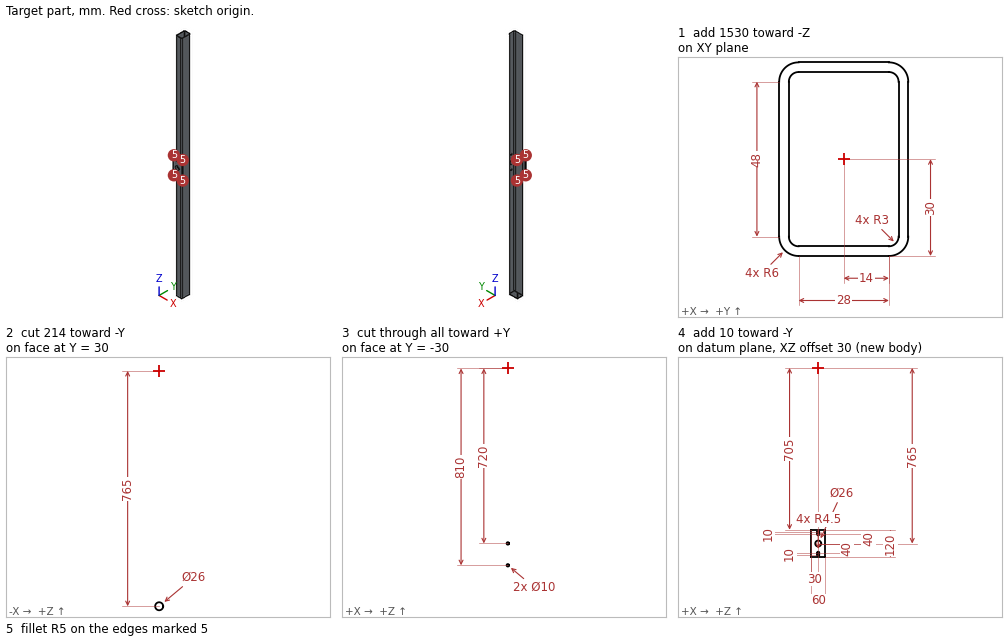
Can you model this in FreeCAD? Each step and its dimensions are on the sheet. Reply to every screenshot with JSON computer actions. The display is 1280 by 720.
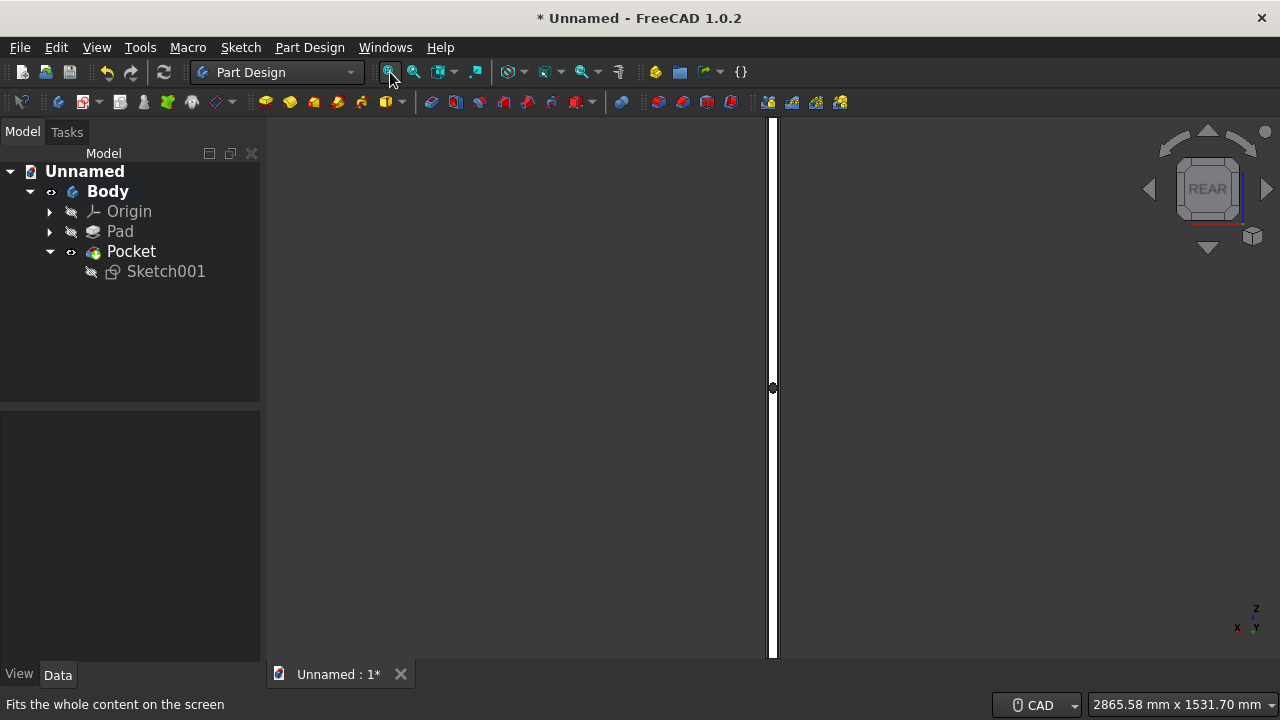
{"action": "key", "text": "0"}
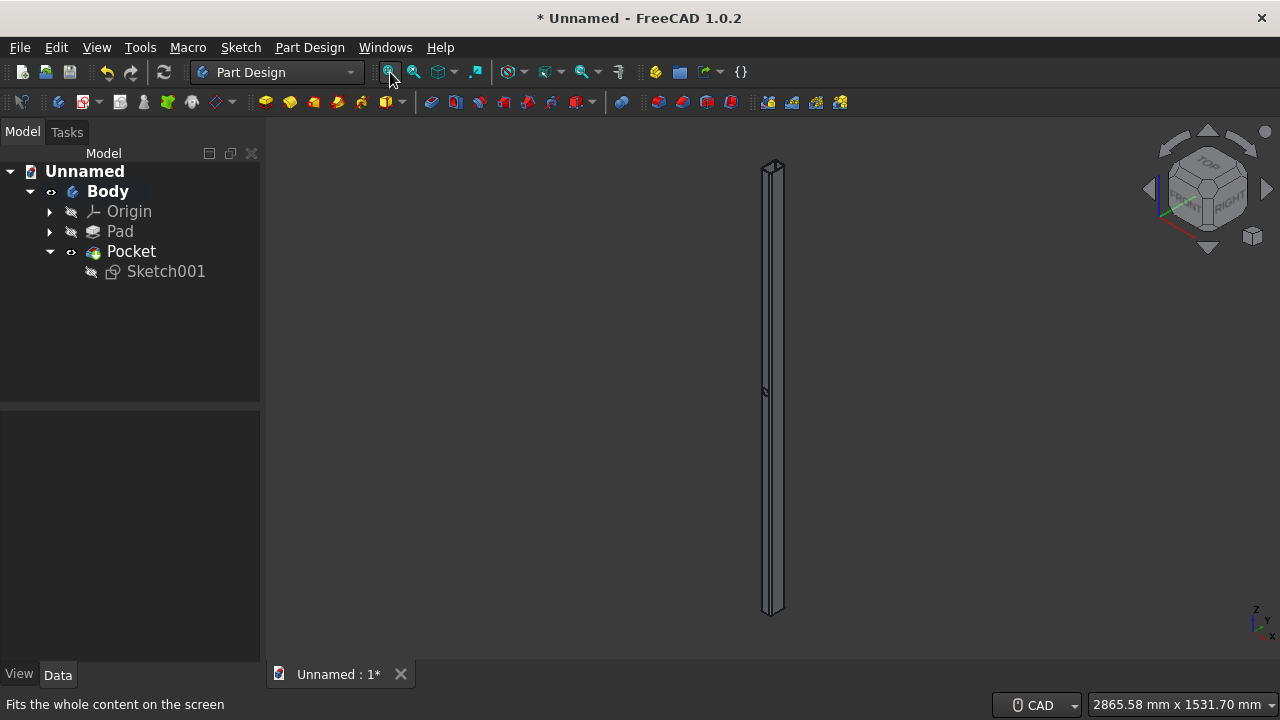
{"action": "scroll", "coordinate": [765, 202], "scroll_direction": "up", "scroll_amount": 5}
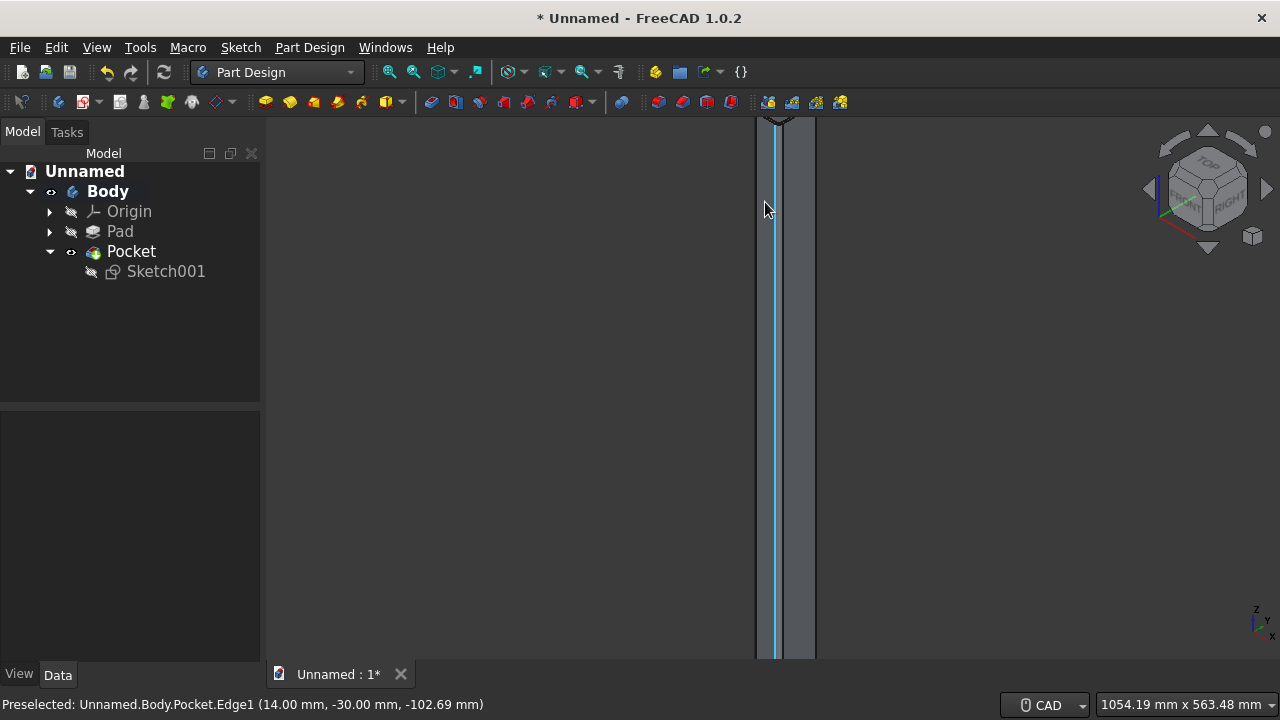
{"action": "left_click", "coordinate": [765, 203]}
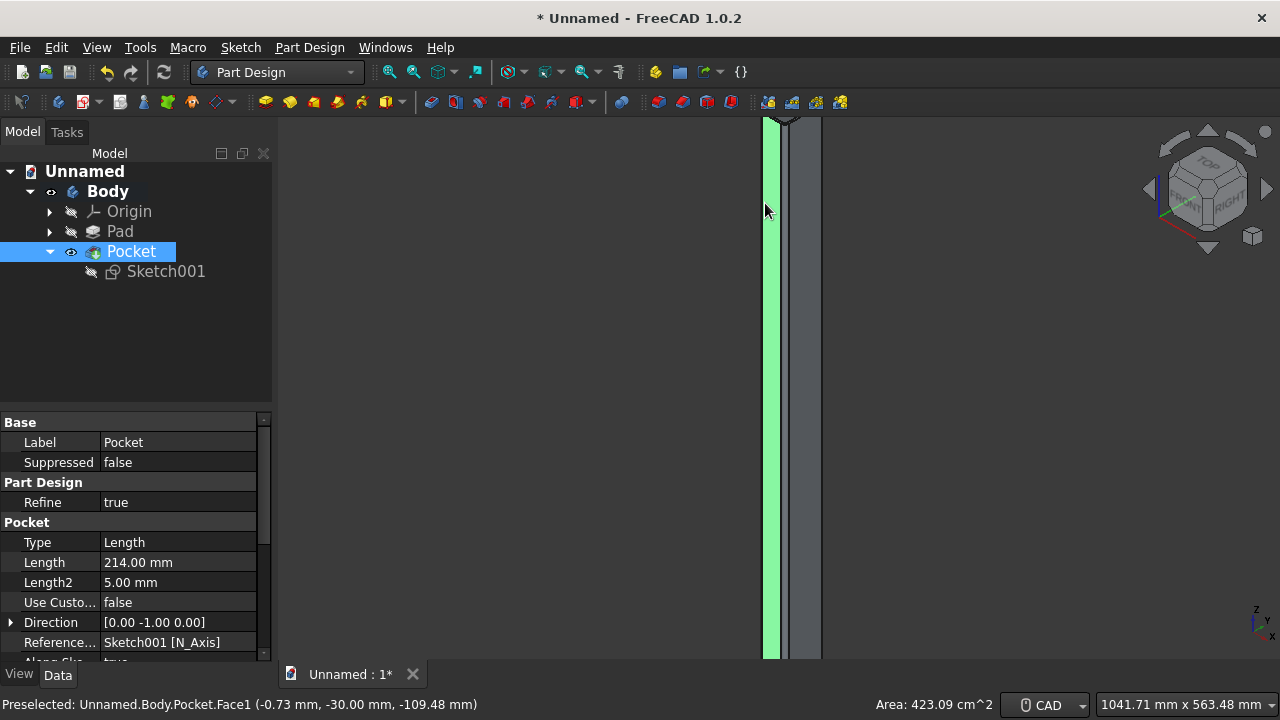
{"action": "left_click", "coordinate": [84, 102]}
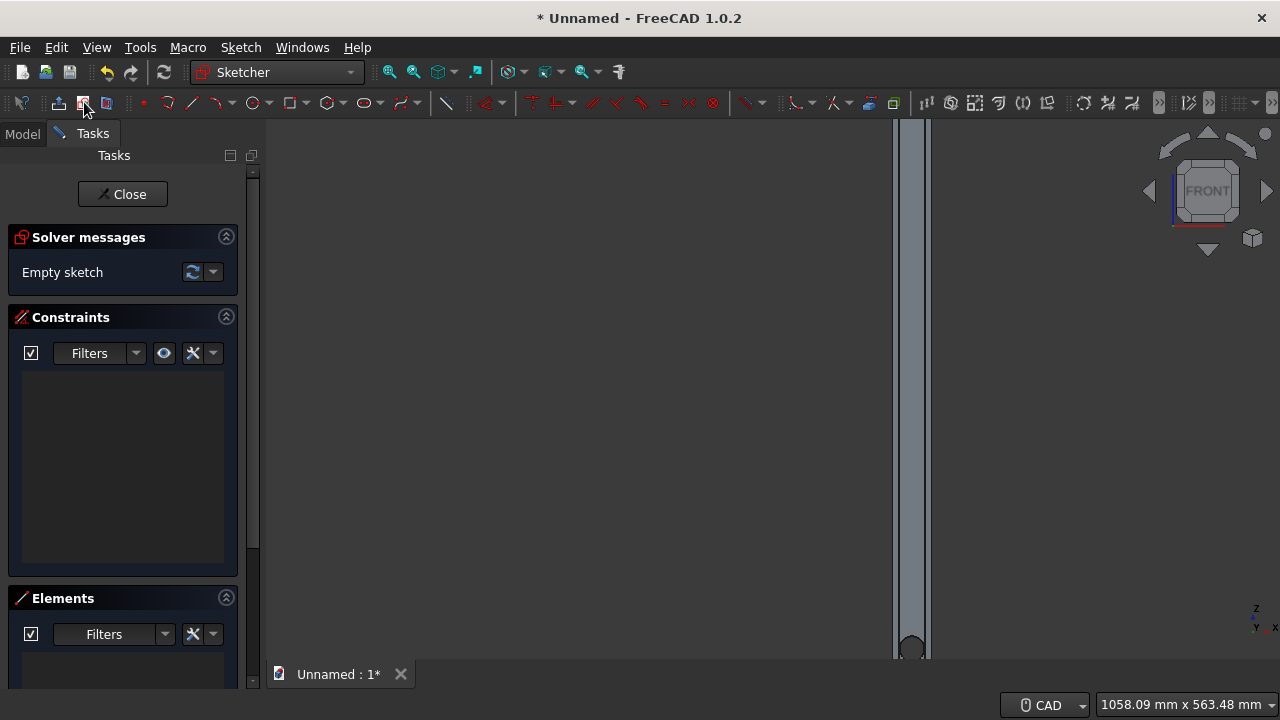
{"action": "scroll", "coordinate": [704, 389], "scroll_direction": "down", "scroll_amount": 5}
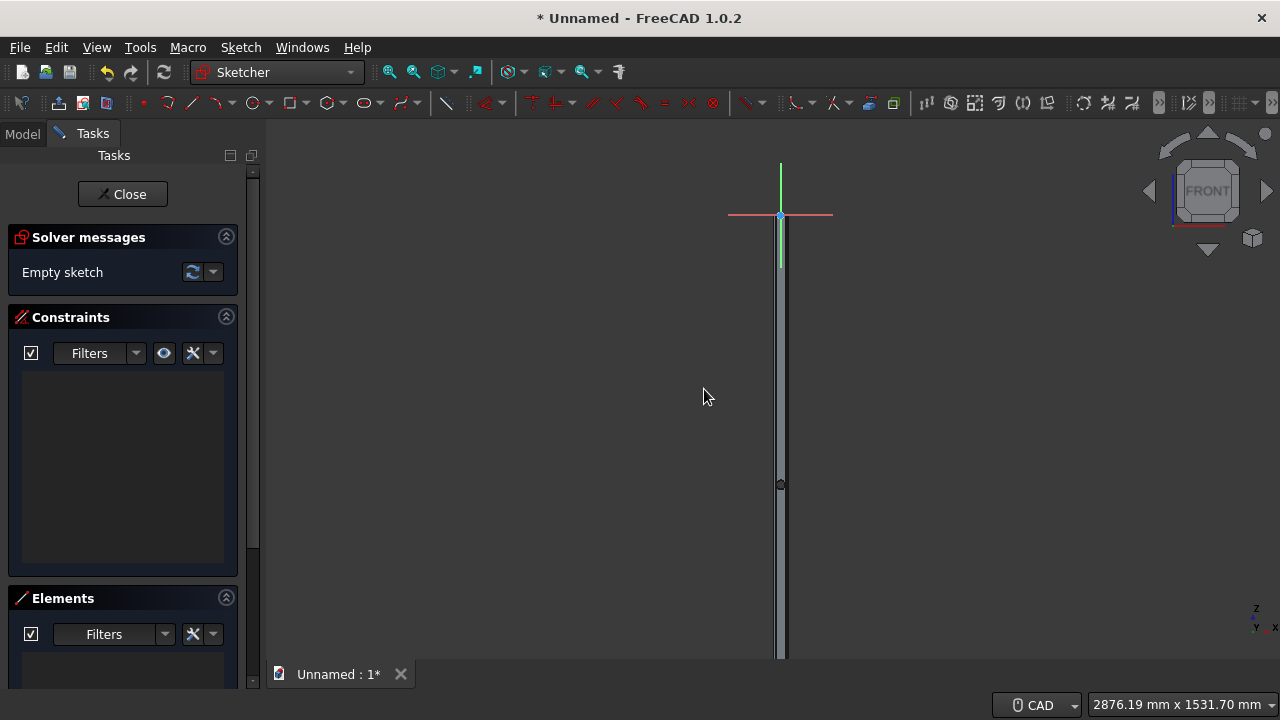
{"action": "scroll", "coordinate": [790, 497], "scroll_direction": "up", "scroll_amount": 11}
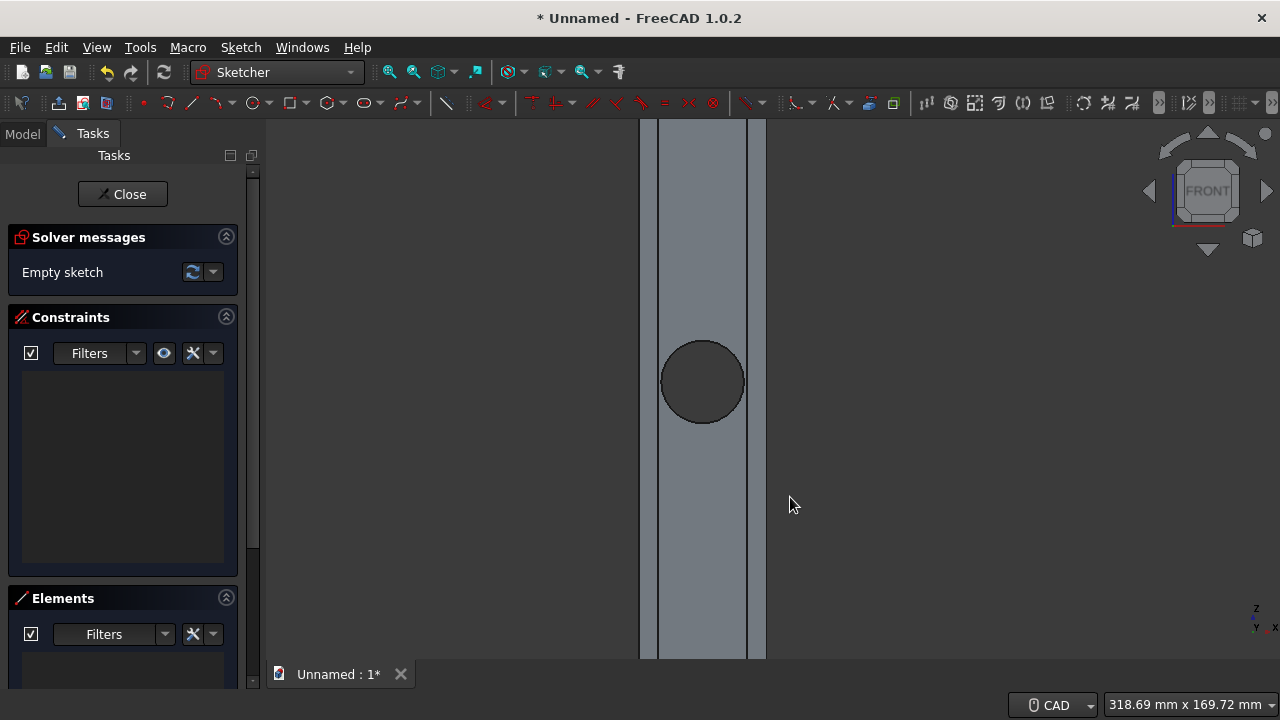
{"action": "left_click", "coordinate": [254, 104]}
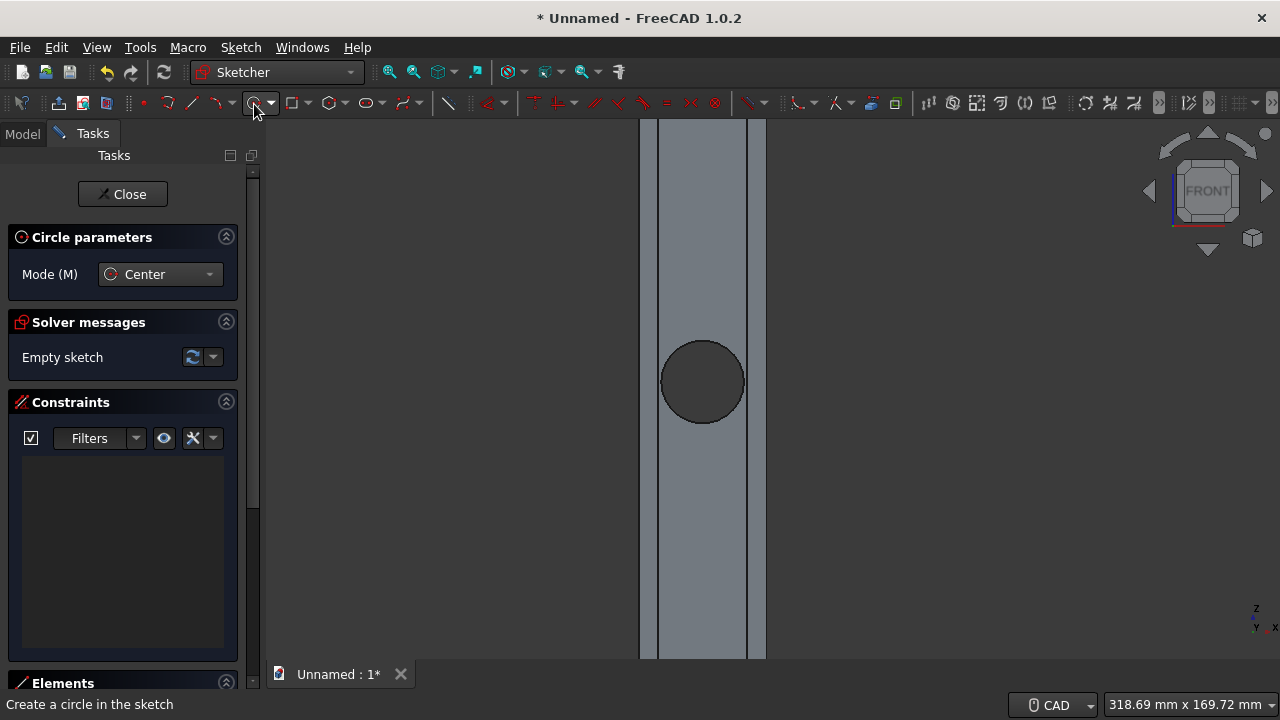
{"action": "scroll", "coordinate": [703, 239], "scroll_direction": "up", "scroll_amount": 2}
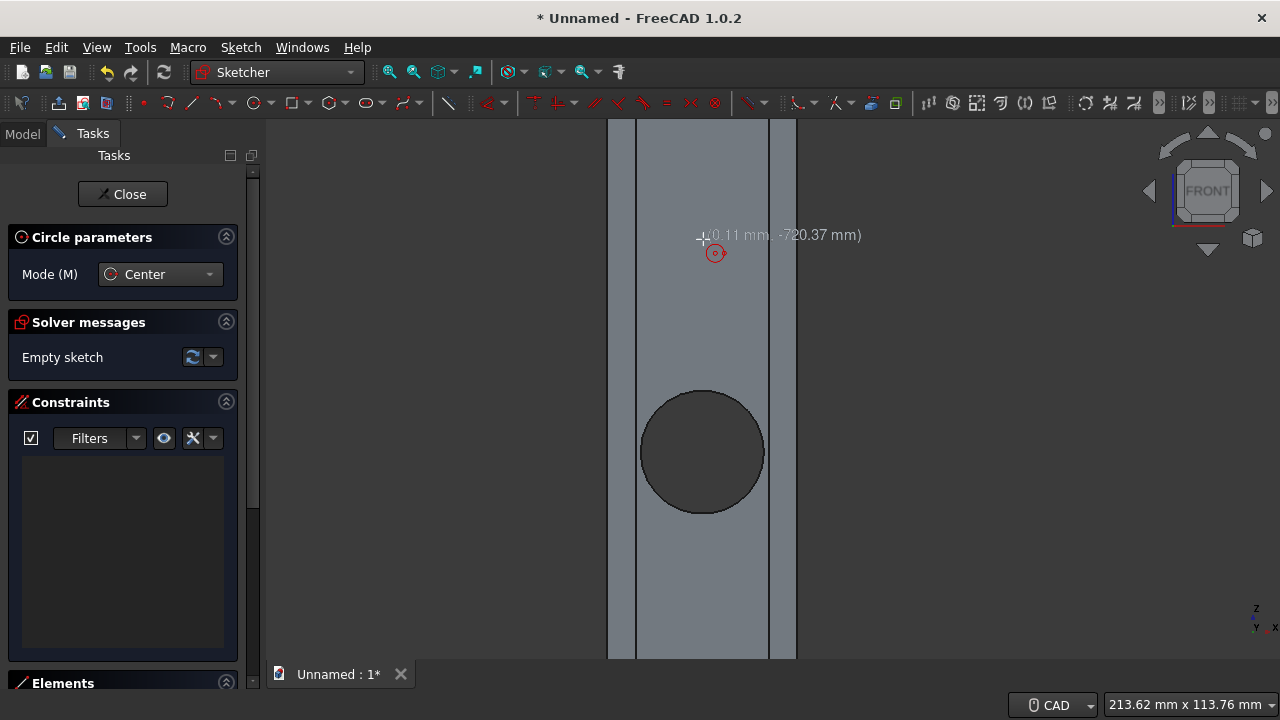
{"action": "left_click", "coordinate": [702, 239]}
{"action": "mouse_move", "coordinate": [719, 222]}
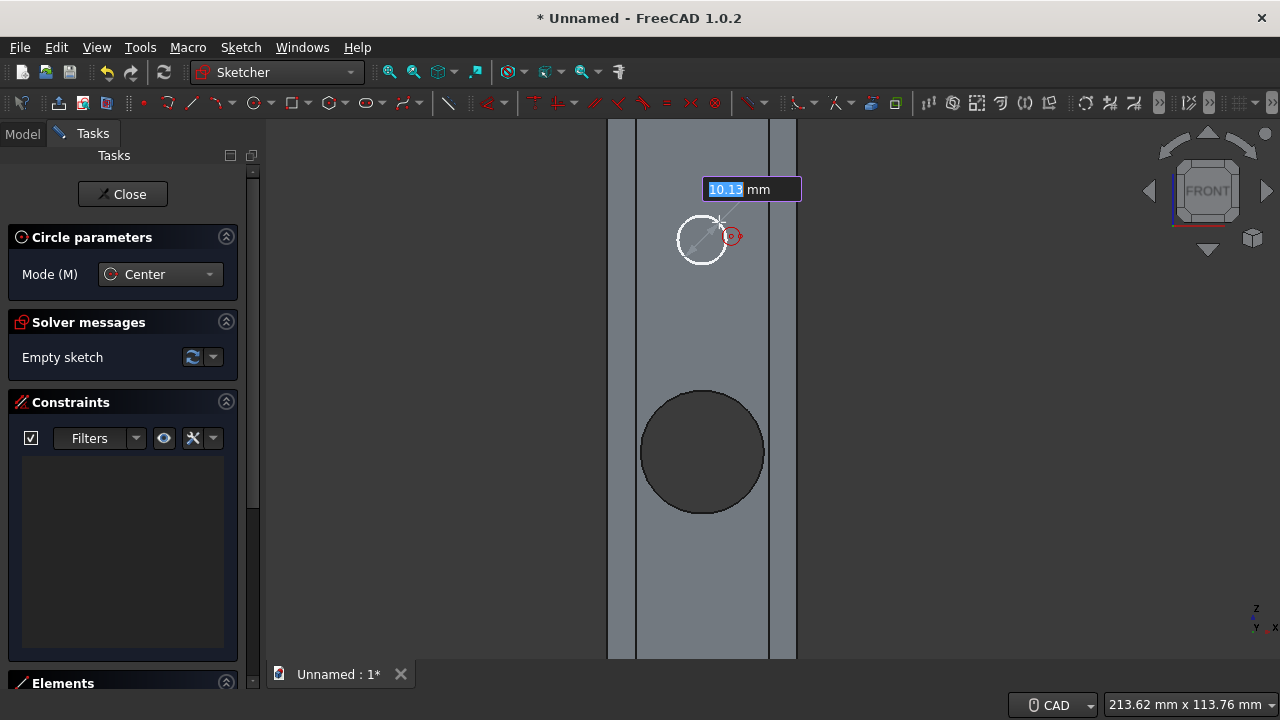
{"action": "type", "text": "10"}
{"action": "key", "text": "Return"}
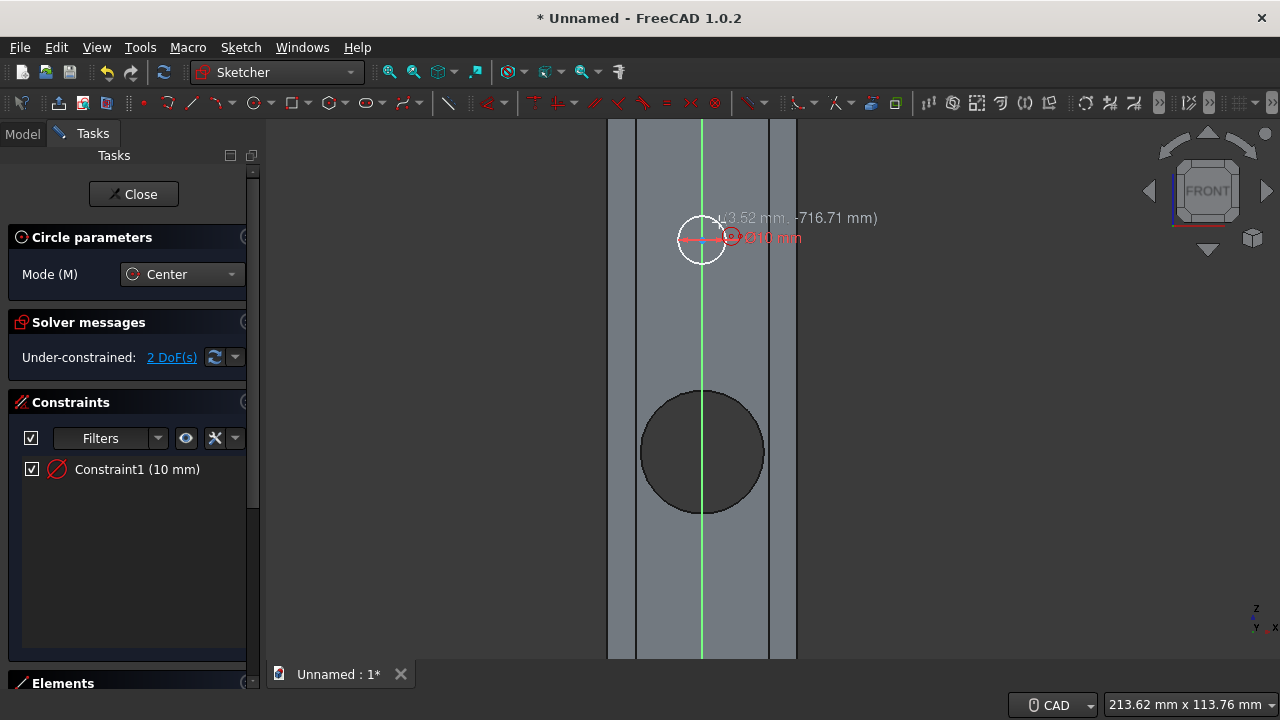
{"action": "scroll", "coordinate": [709, 260], "scroll_direction": "down", "scroll_amount": 2}